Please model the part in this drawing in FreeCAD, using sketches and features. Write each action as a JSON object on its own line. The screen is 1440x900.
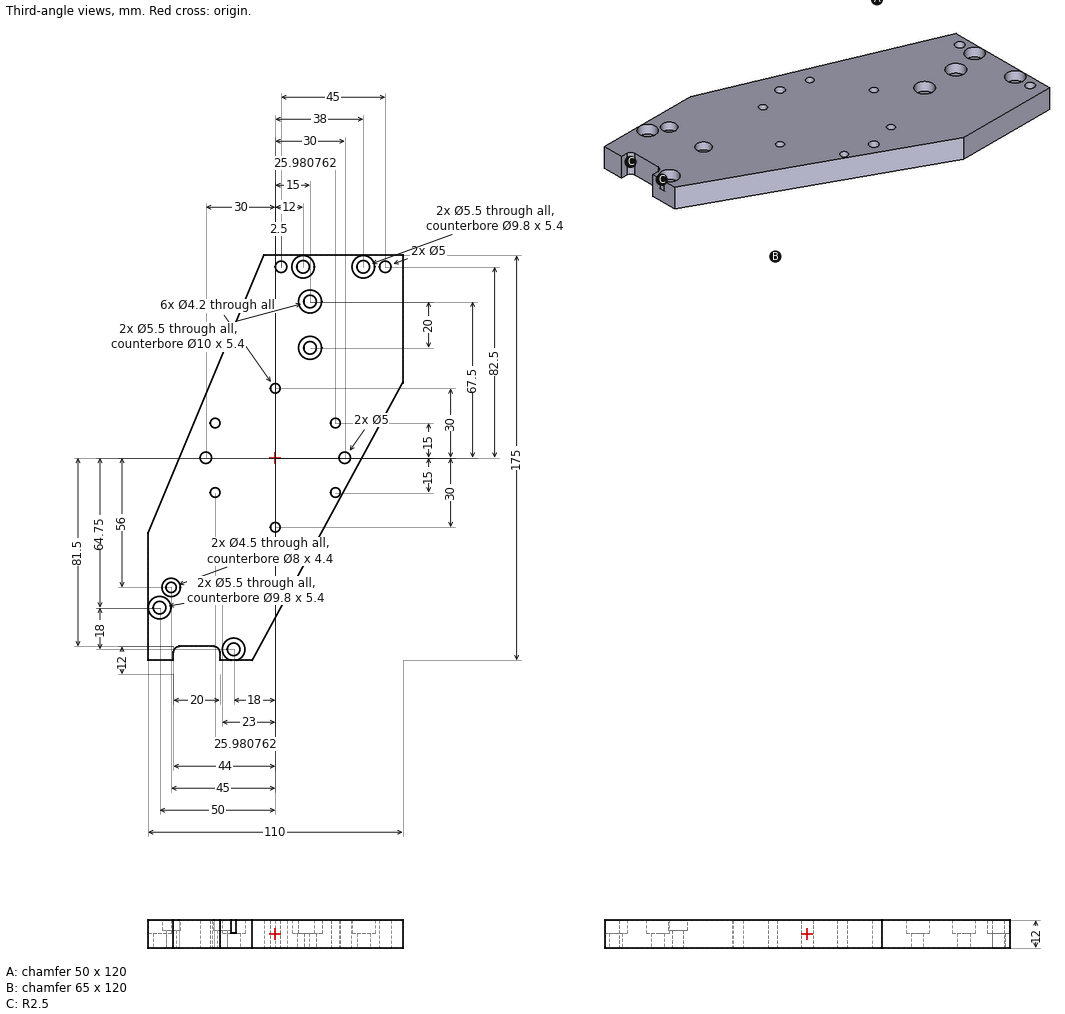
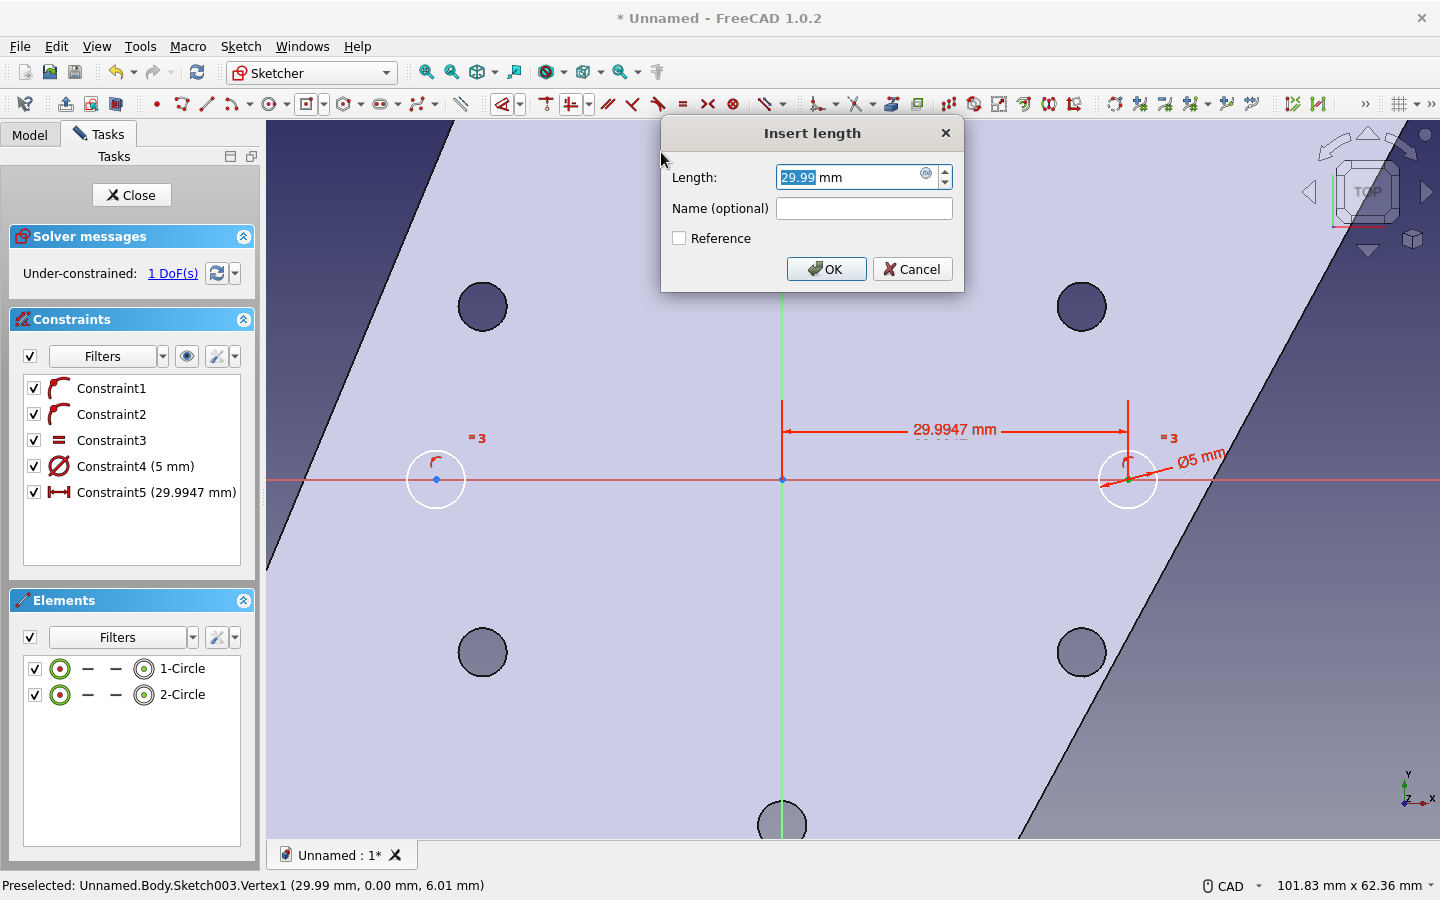
{"action": "type", "text": "30"}
{"action": "key", "text": "Return"}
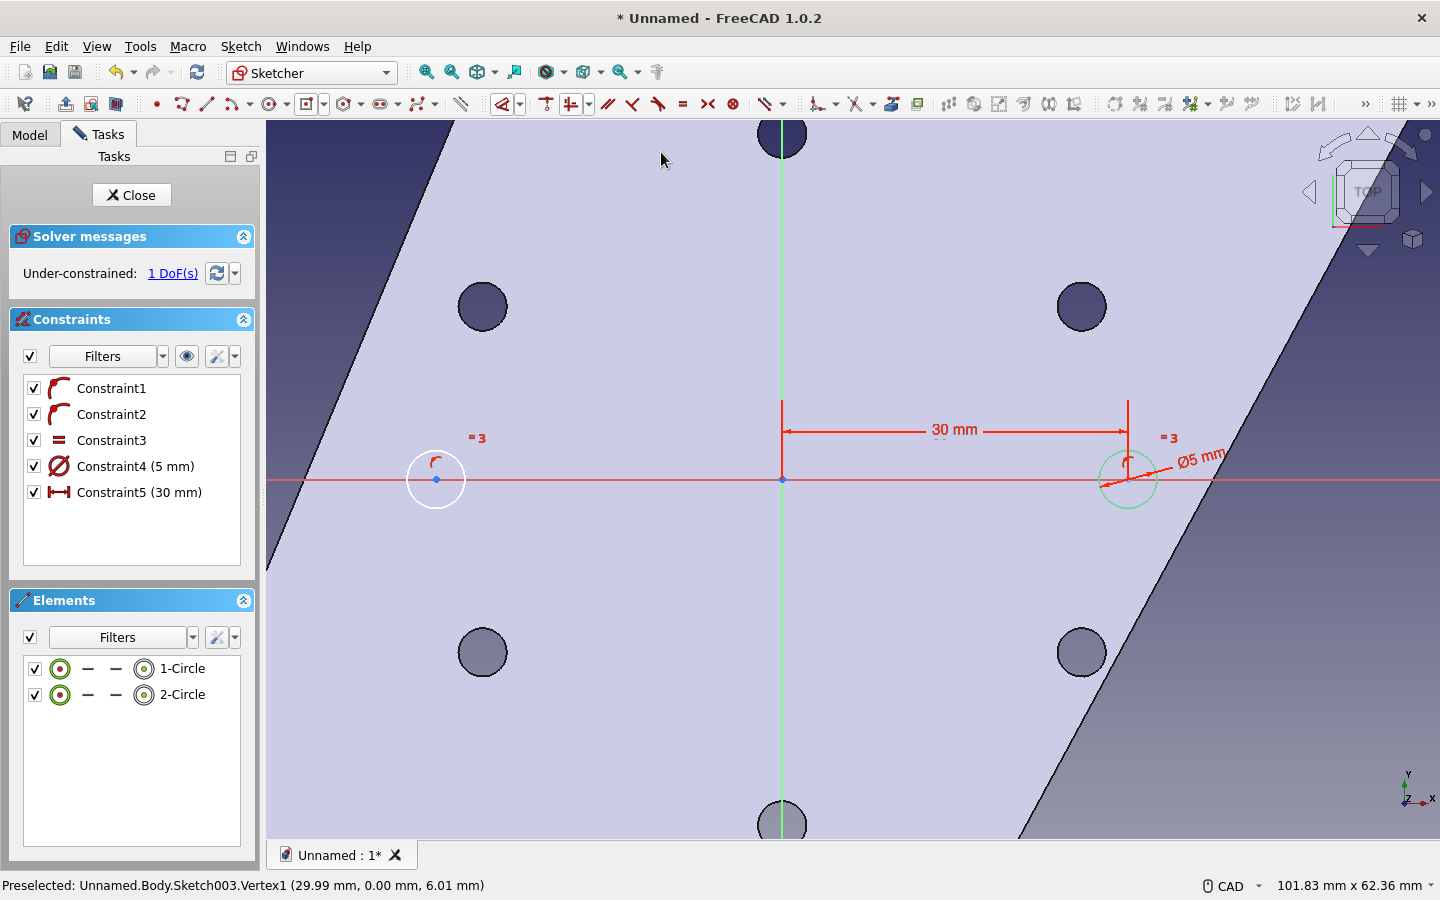
{"action": "left_click", "coordinate": [436, 479]}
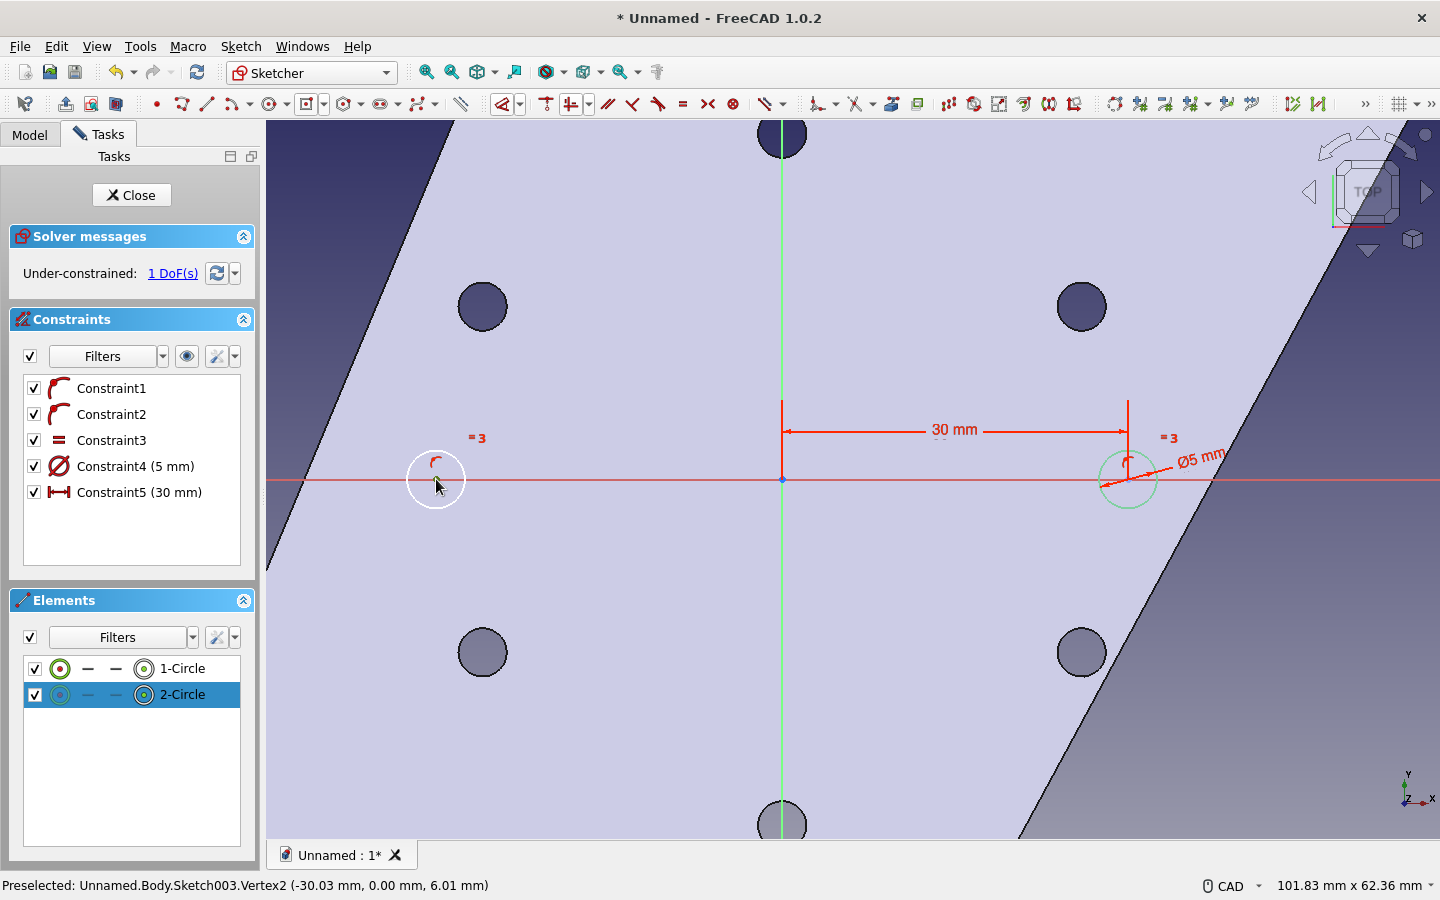
{"action": "key", "text": "l"}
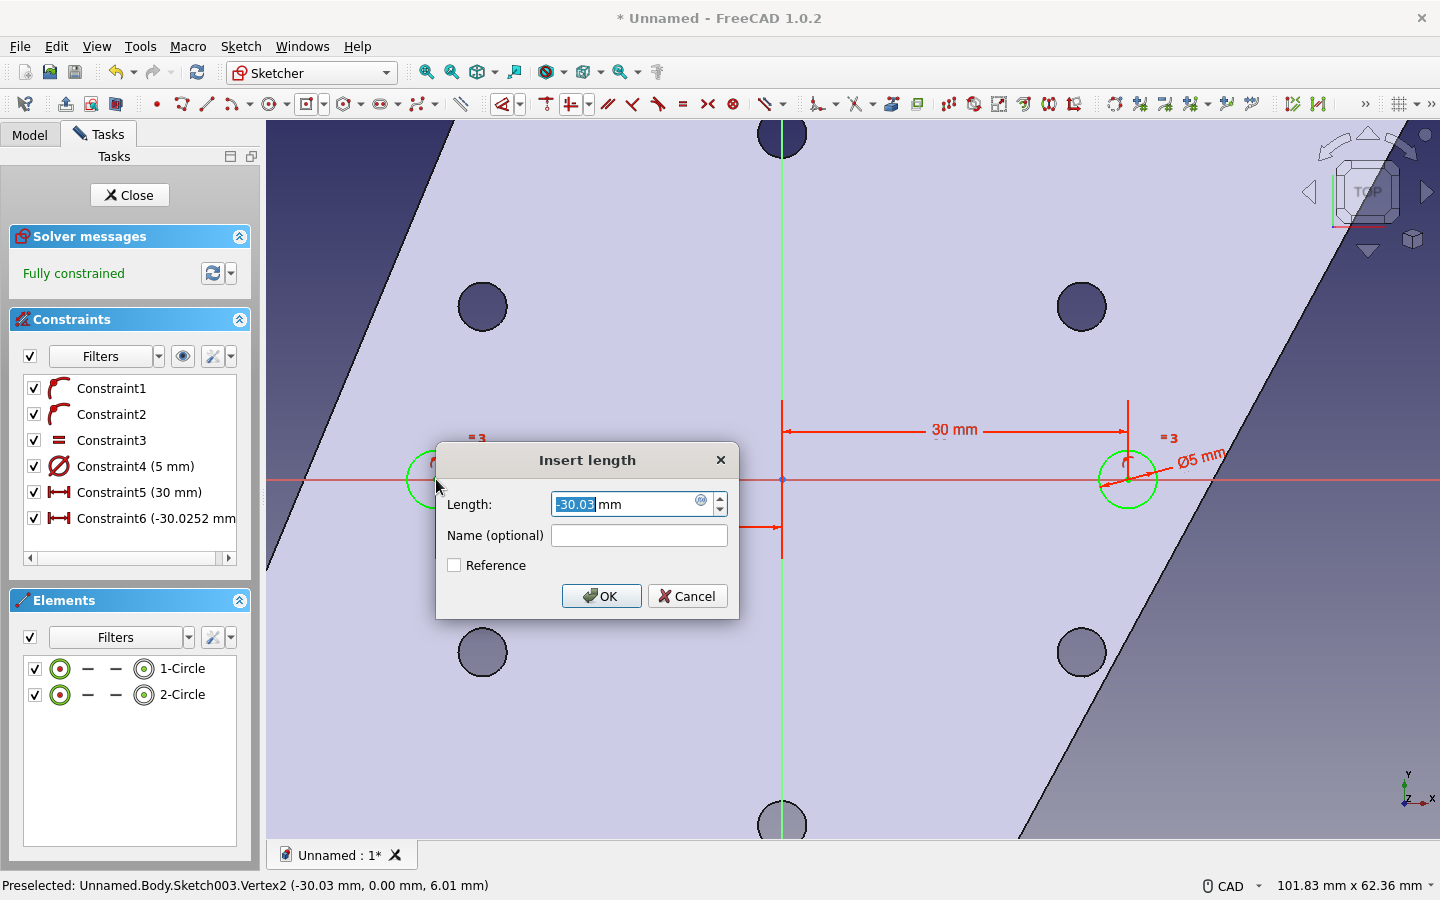
{"action": "type", "text": "-30"}
{"action": "key", "text": "Return"}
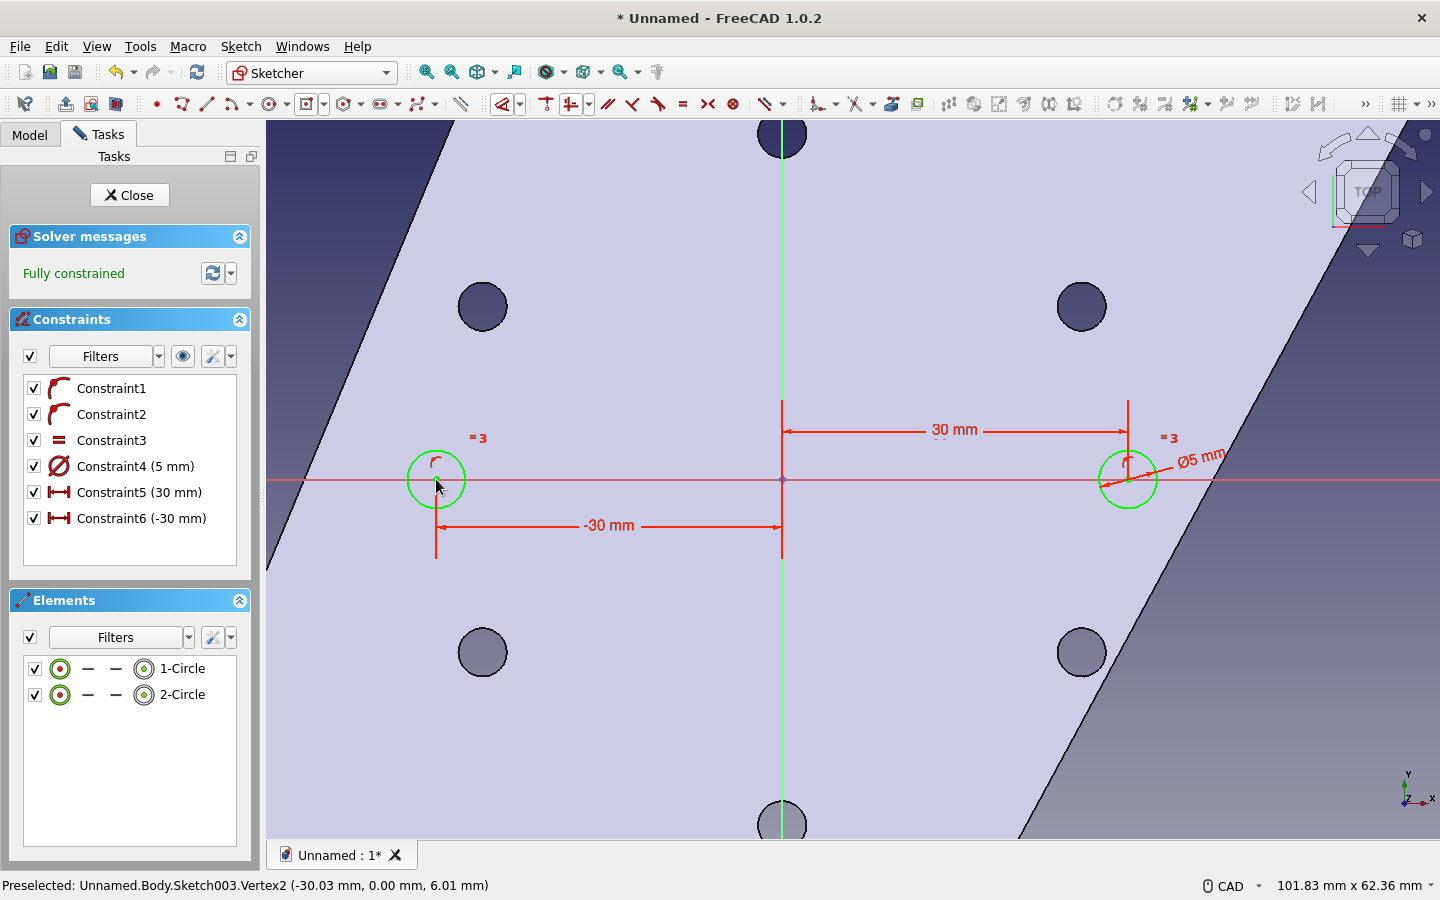
{"action": "left_click", "coordinate": [130, 195]}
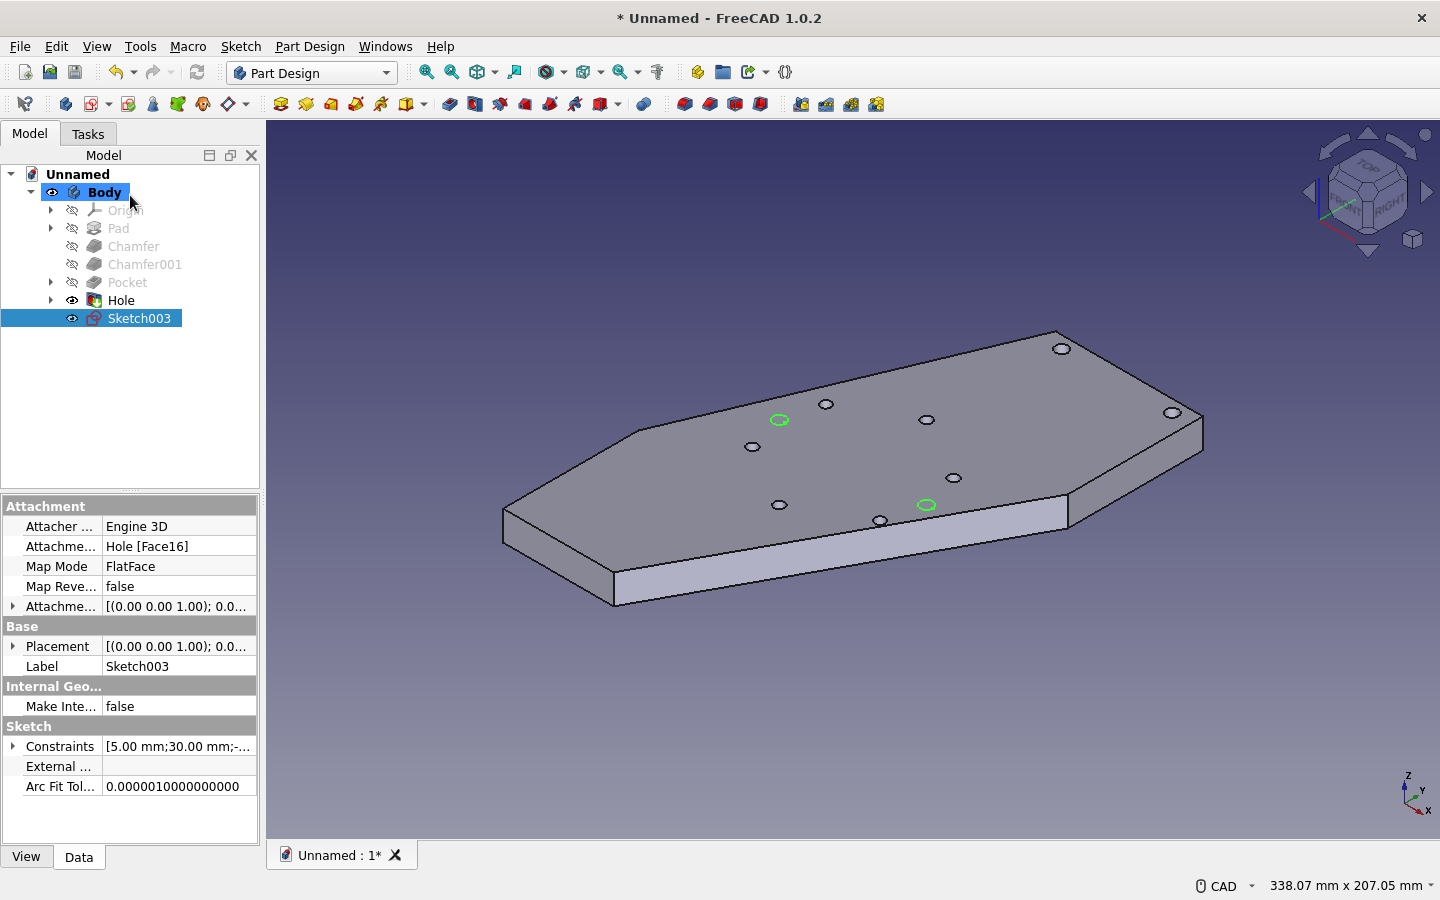
{"action": "left_click", "coordinate": [450, 104]}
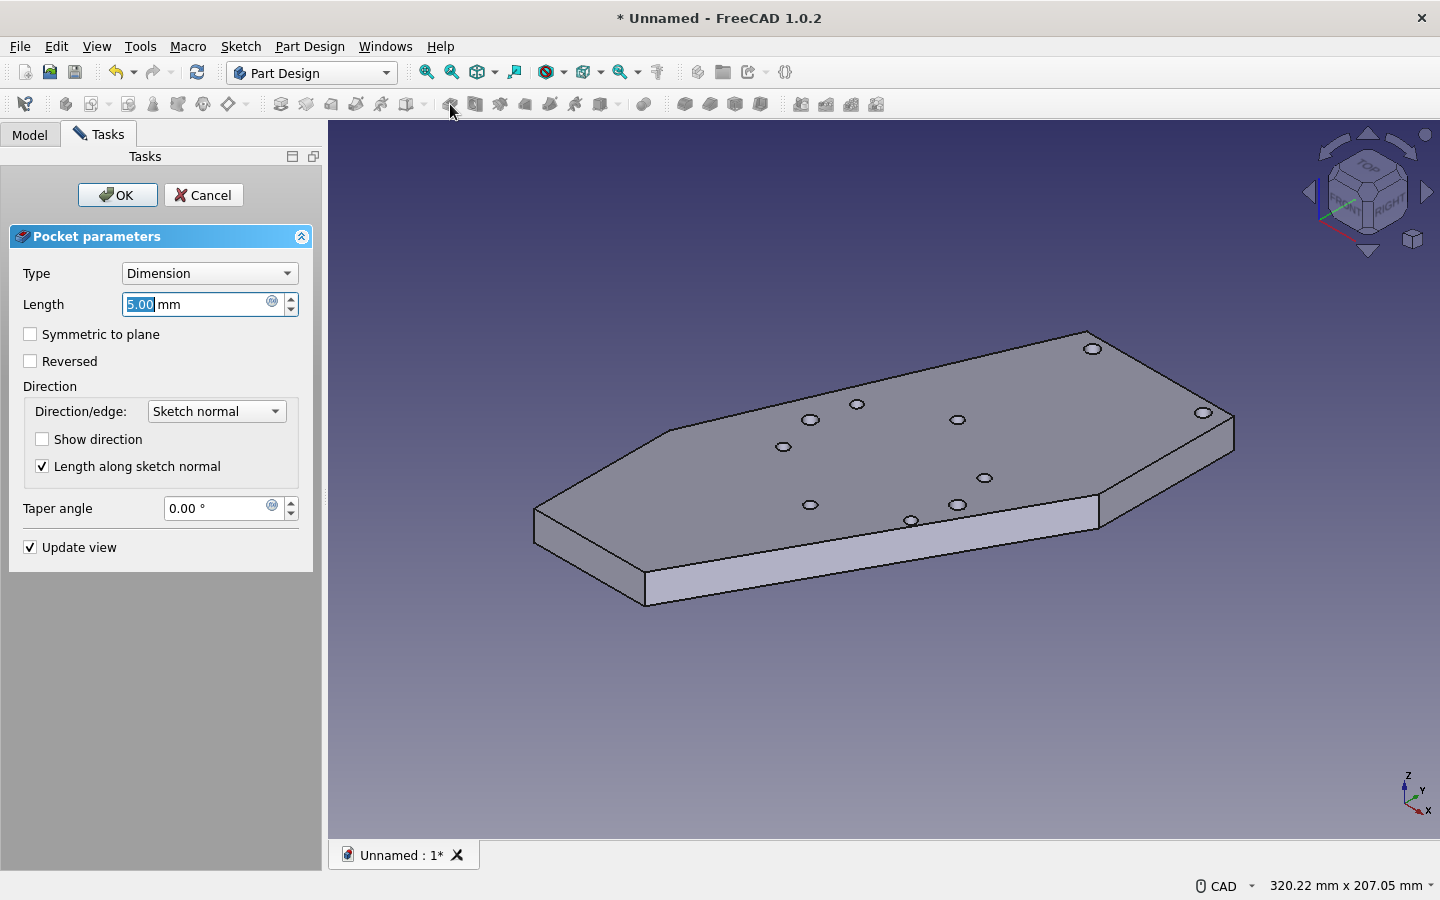
{"action": "left_click", "coordinate": [210, 274]}